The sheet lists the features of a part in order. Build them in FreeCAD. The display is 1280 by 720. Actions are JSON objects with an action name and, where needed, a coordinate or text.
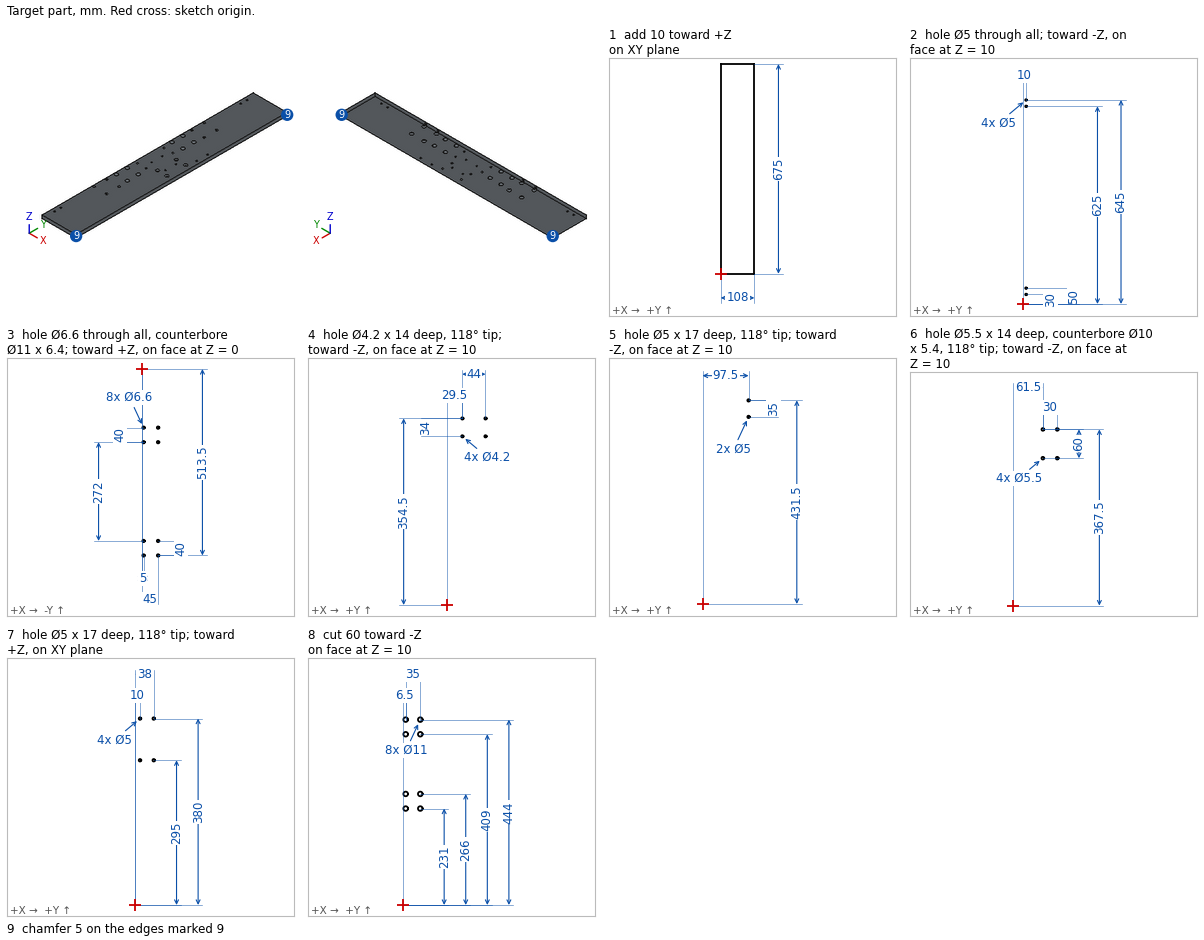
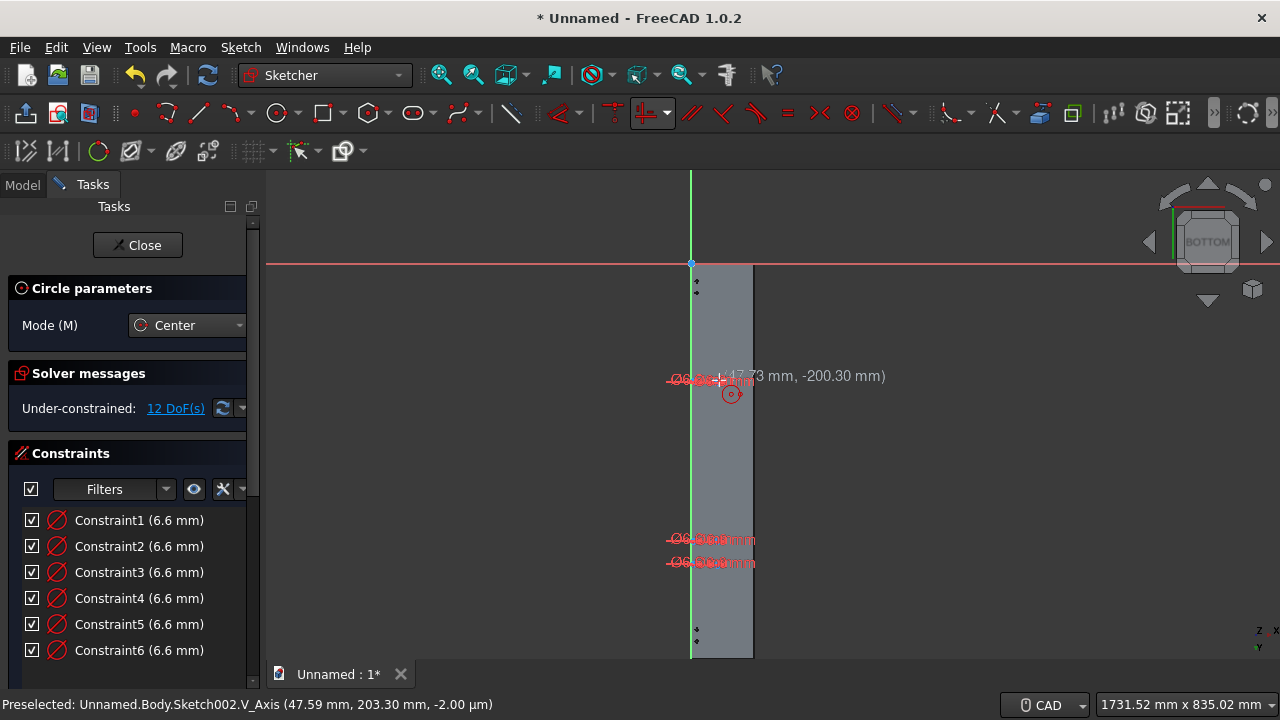
{"action": "scroll", "coordinate": [694, 358], "scroll_direction": "up", "scroll_amount": 13}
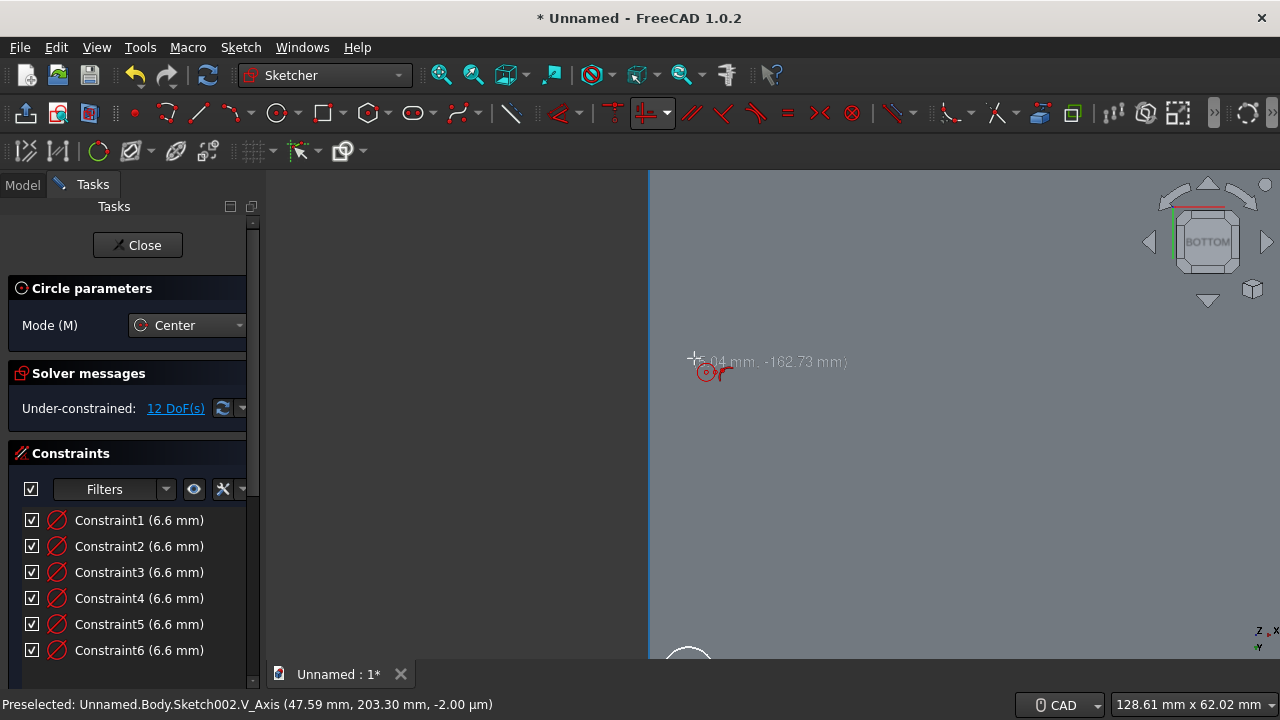
{"action": "left_click", "coordinate": [688, 357]}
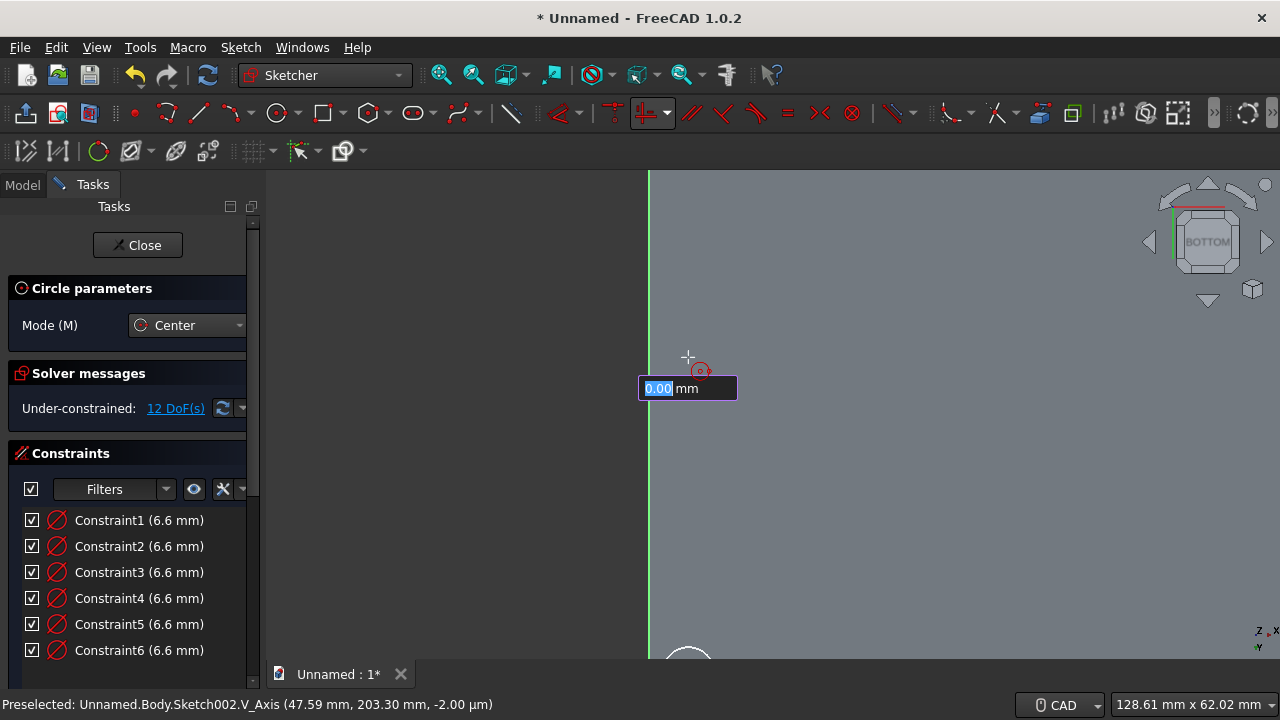
{"action": "scroll", "coordinate": [694, 358], "scroll_direction": "down", "scroll_amount": 13}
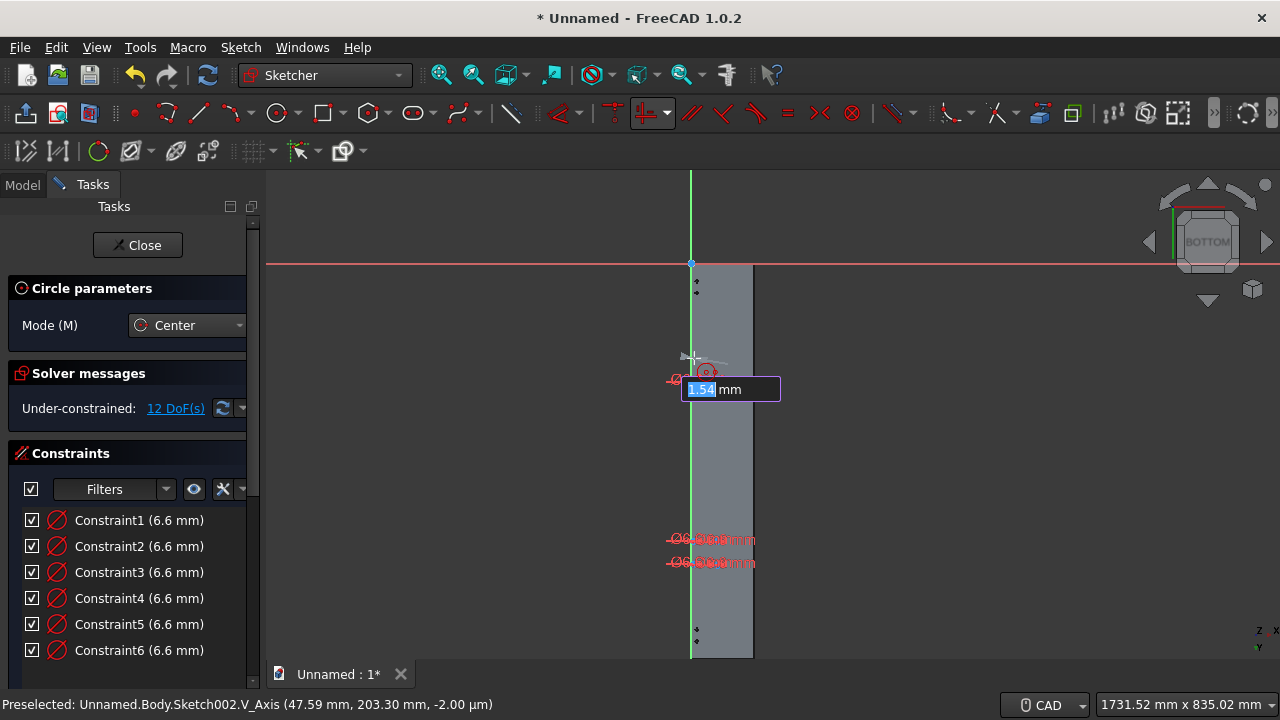
{"action": "scroll", "coordinate": [695, 357], "scroll_direction": "up", "scroll_amount": 7}
{"action": "mouse_move", "coordinate": [695, 355]}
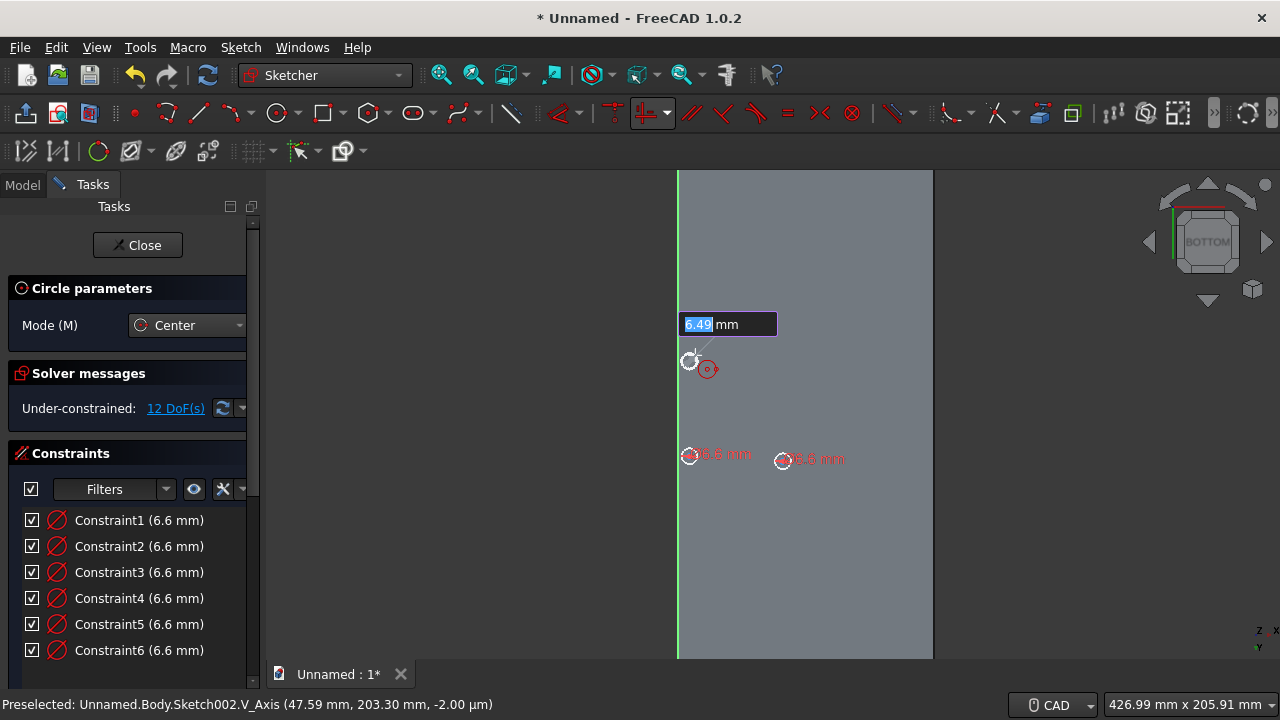
{"action": "type", "text": "6.6"}
{"action": "key", "text": "Return"}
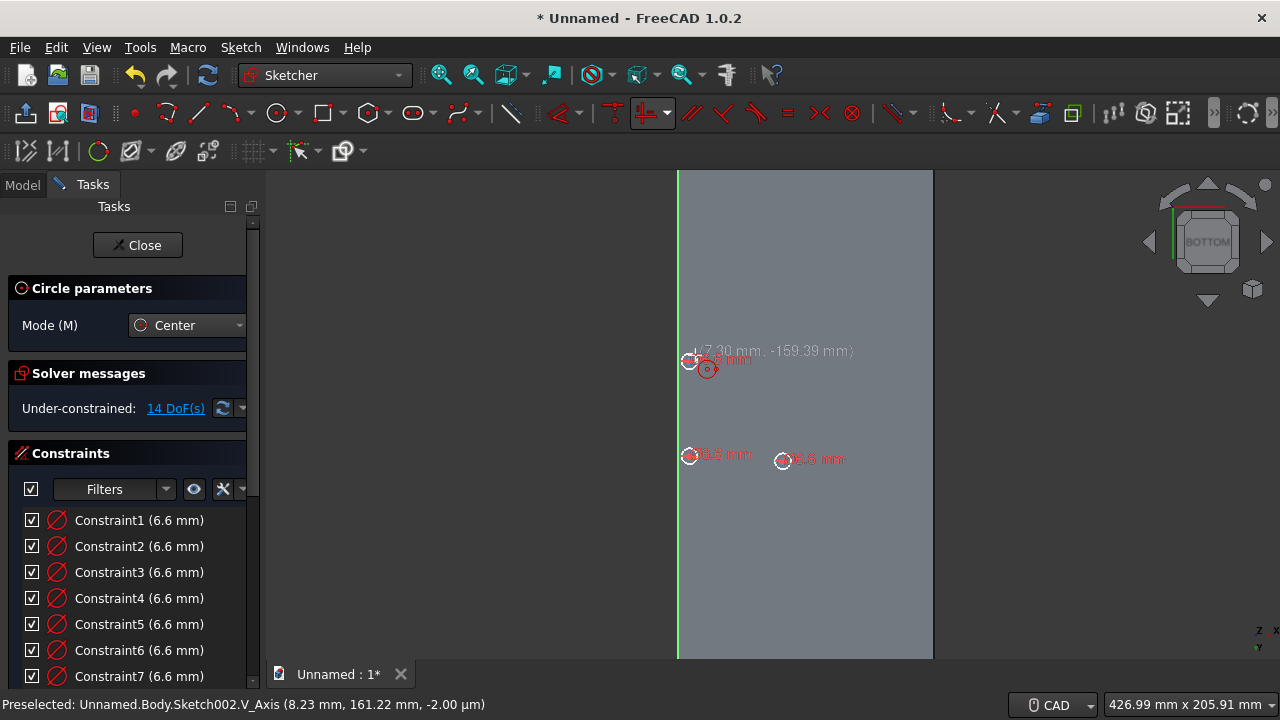
{"action": "scroll", "coordinate": [785, 361], "scroll_direction": "up", "scroll_amount": 6}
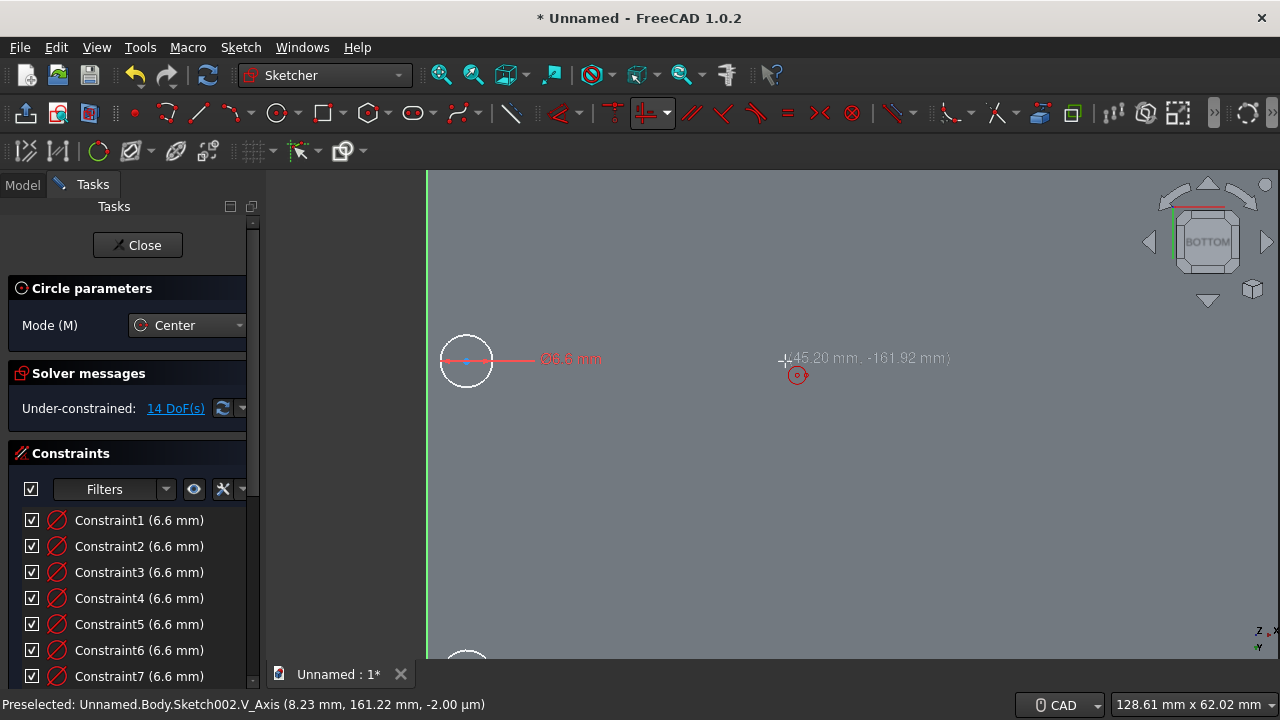
{"action": "scroll", "coordinate": [711, 358], "scroll_direction": "down", "scroll_amount": 13}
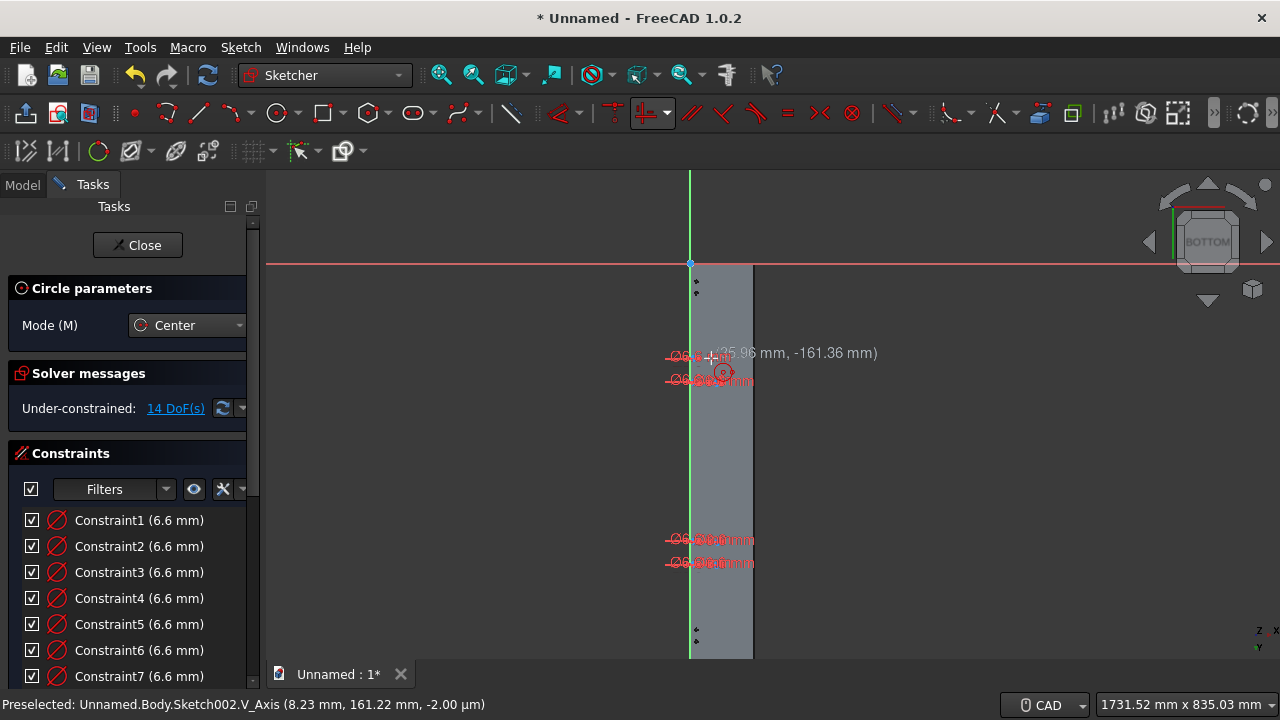
{"action": "left_click", "coordinate": [717, 359]}
{"action": "mouse_move", "coordinate": [718, 357]}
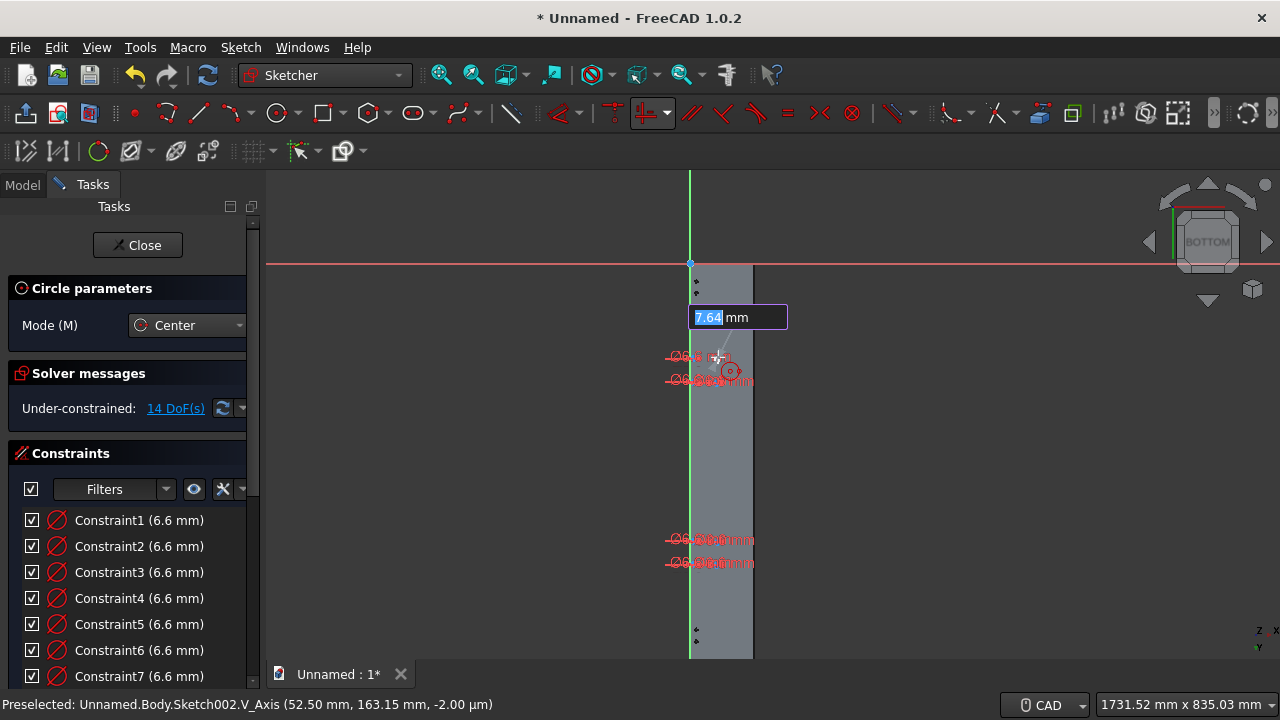
{"action": "type", "text": "6.6"}
{"action": "key", "text": "Return"}
{"action": "key", "text": "Escape"}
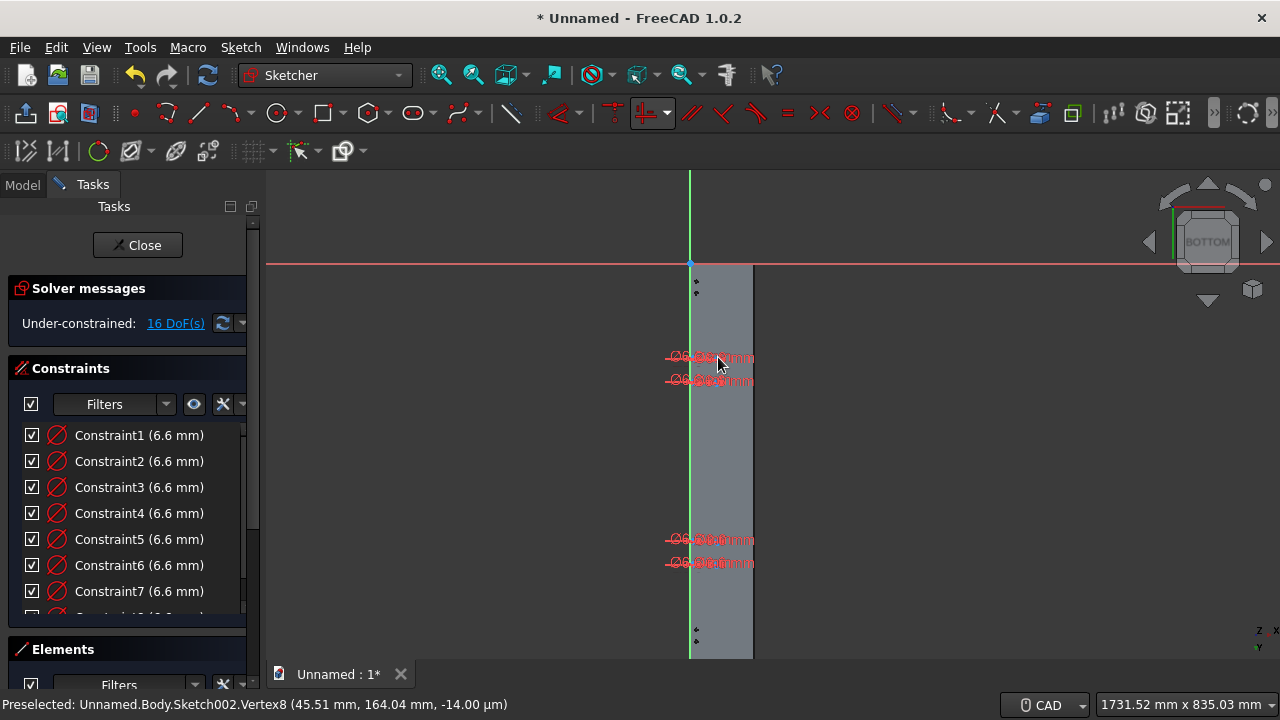
{"action": "left_click", "coordinate": [717, 565]}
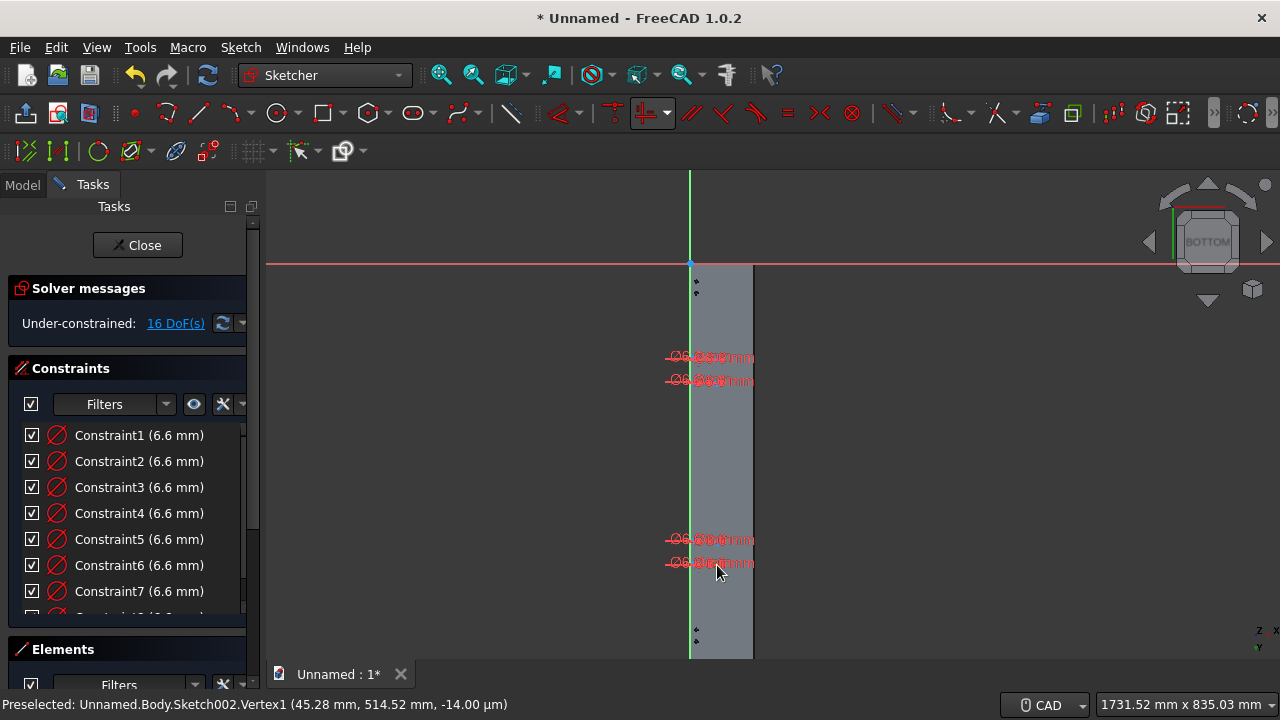
{"action": "left_click", "coordinate": [693, 565]}